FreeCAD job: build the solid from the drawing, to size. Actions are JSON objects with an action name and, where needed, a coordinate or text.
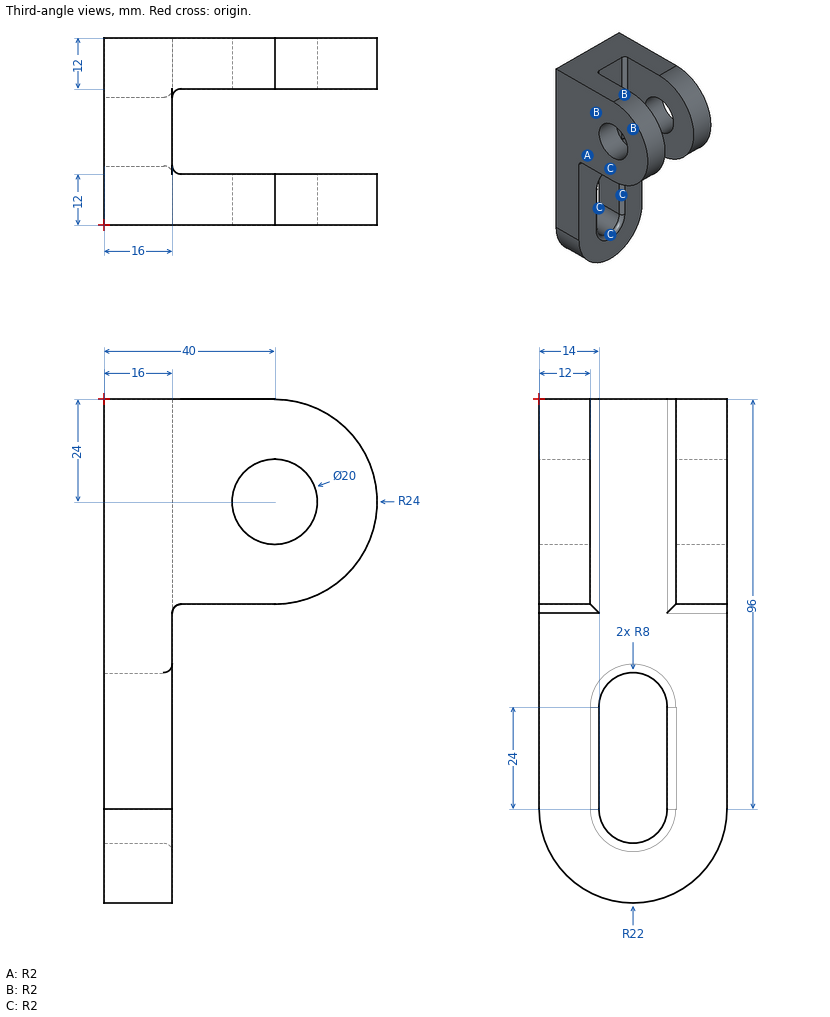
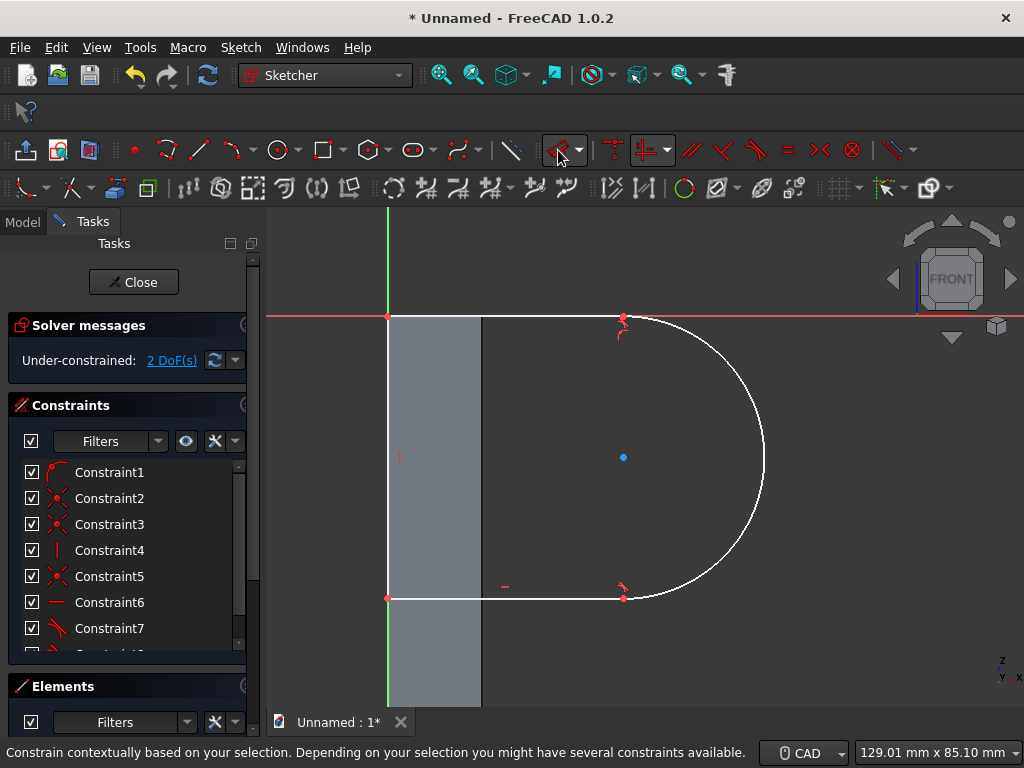
{"action": "left_click", "coordinate": [737, 541]}
{"action": "left_click", "coordinate": [763, 560]}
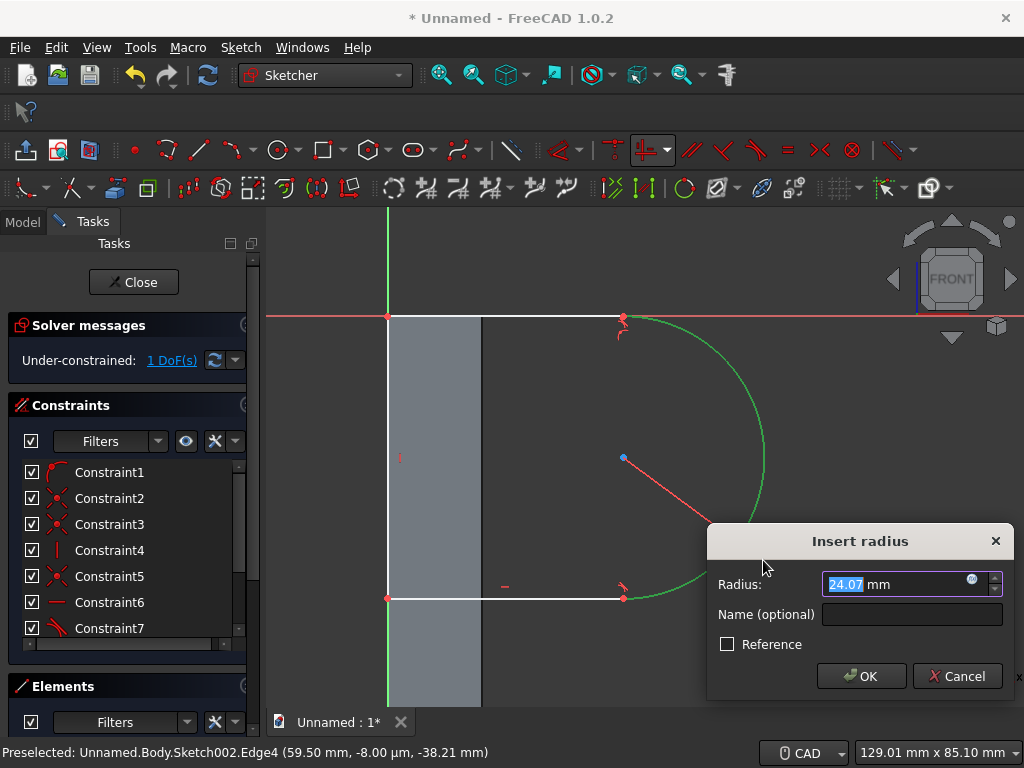
{"action": "type", "text": "24"}
{"action": "key", "text": "Return"}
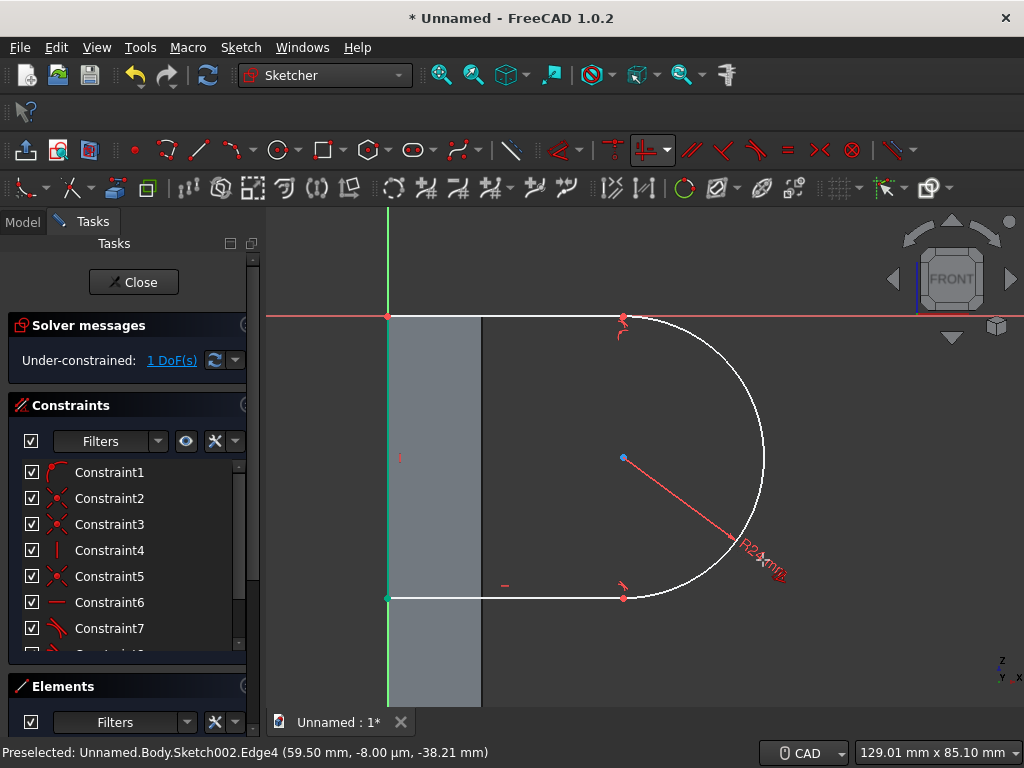
{"action": "left_click", "coordinate": [552, 316]}
{"action": "left_click", "coordinate": [505, 282]}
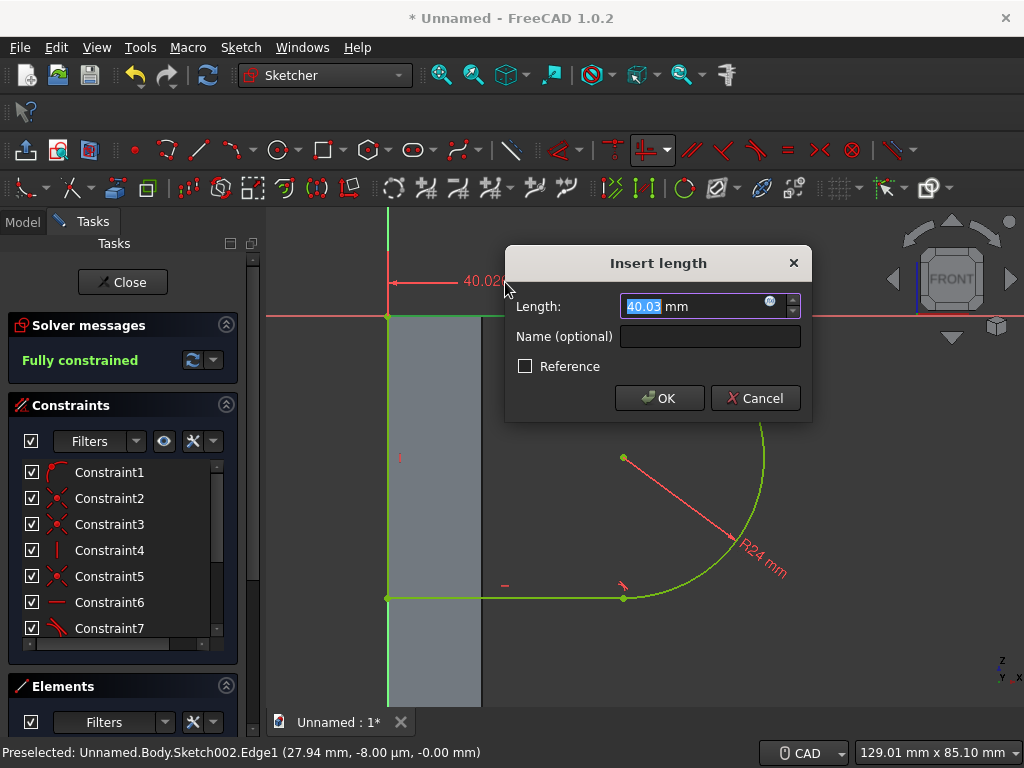
{"action": "type", "text": "40"}
{"action": "key", "text": "Return"}
{"action": "key", "text": "Escape"}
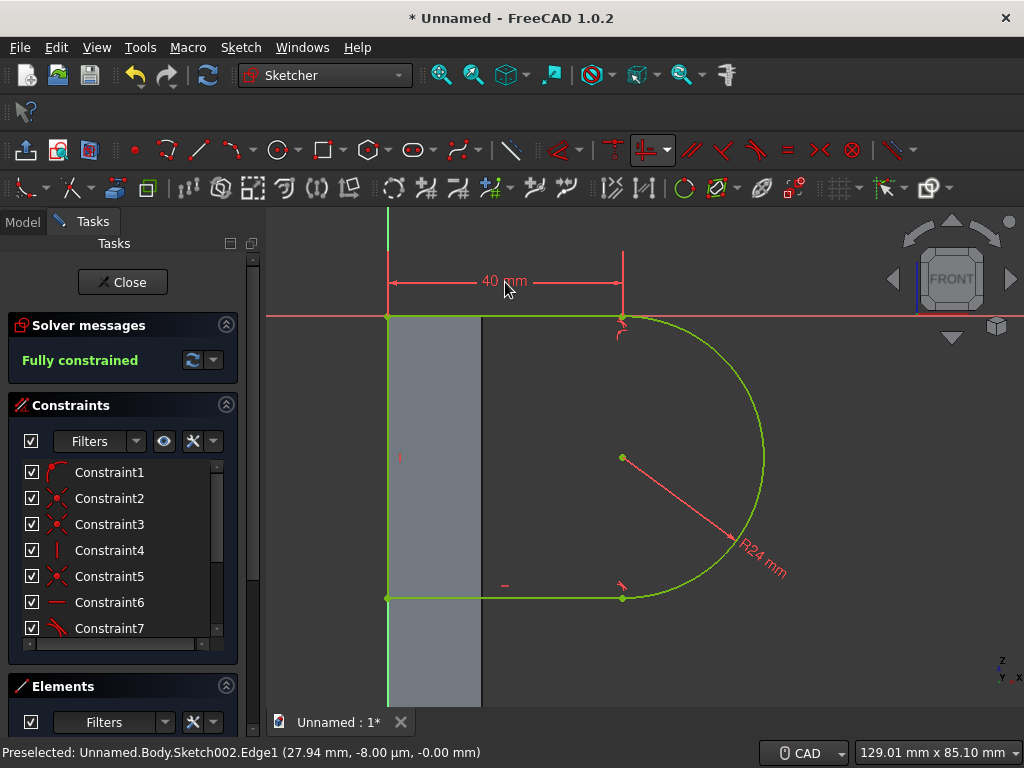
{"action": "left_click", "coordinate": [123, 282]}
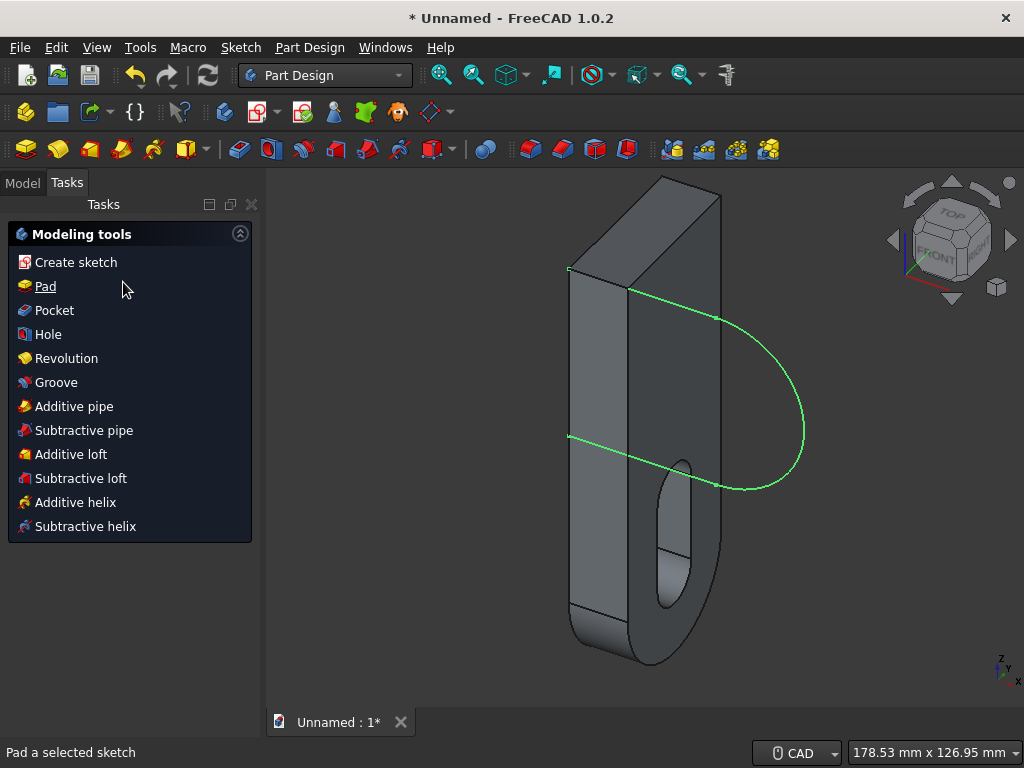
{"action": "left_click", "coordinate": [26, 150]}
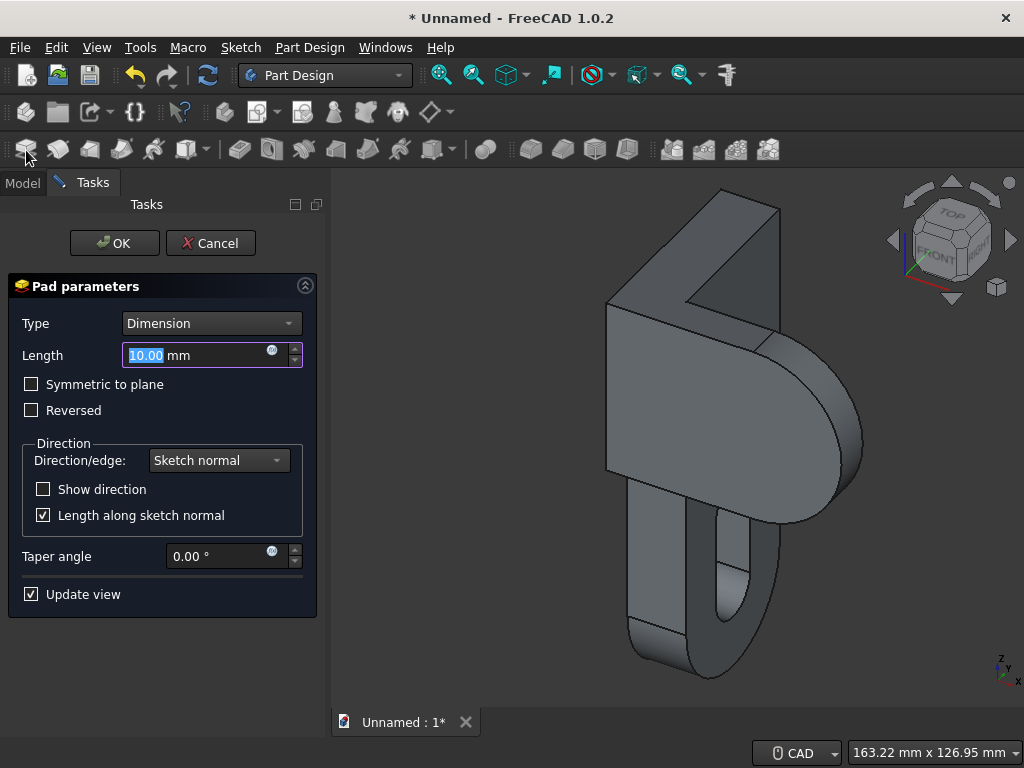
{"action": "type", "text": "12"}
{"action": "key", "text": "Tab"}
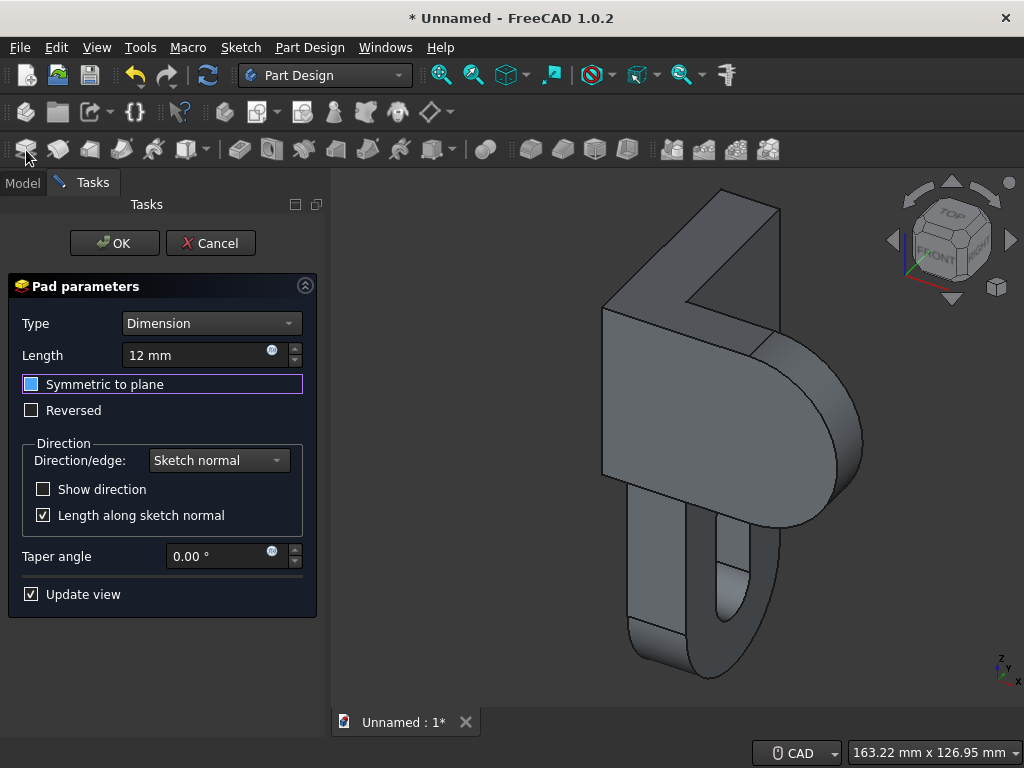
{"action": "left_click", "coordinate": [30, 410]}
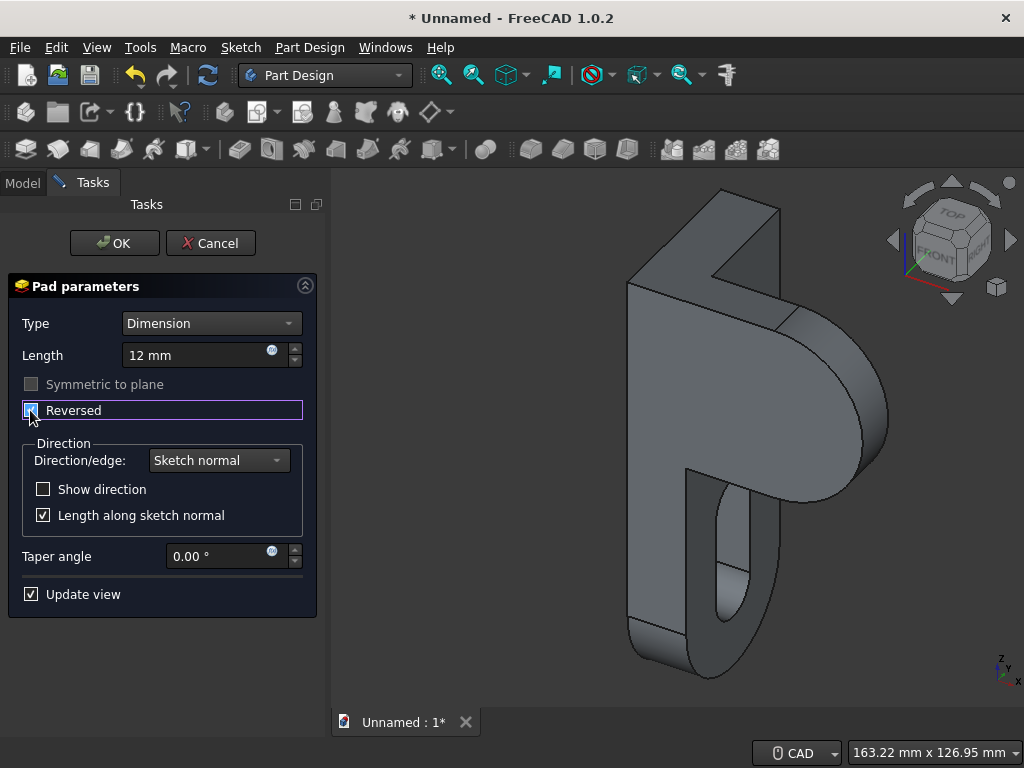
{"action": "left_click", "coordinate": [115, 243]}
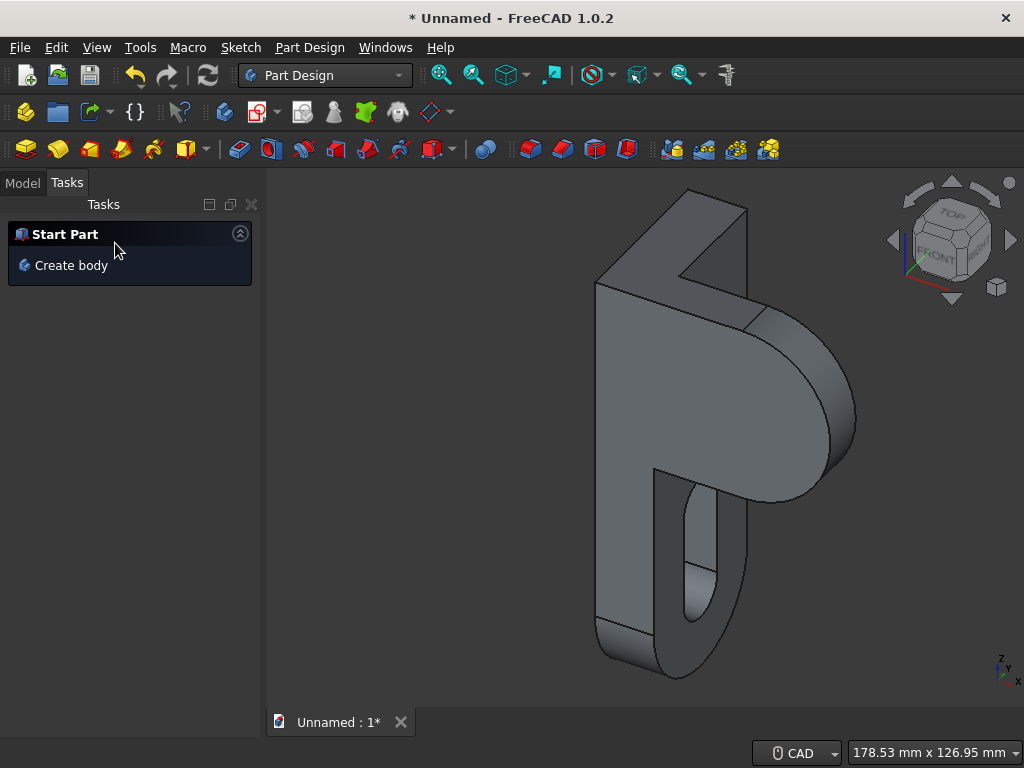
{"action": "left_click", "coordinate": [442, 76]}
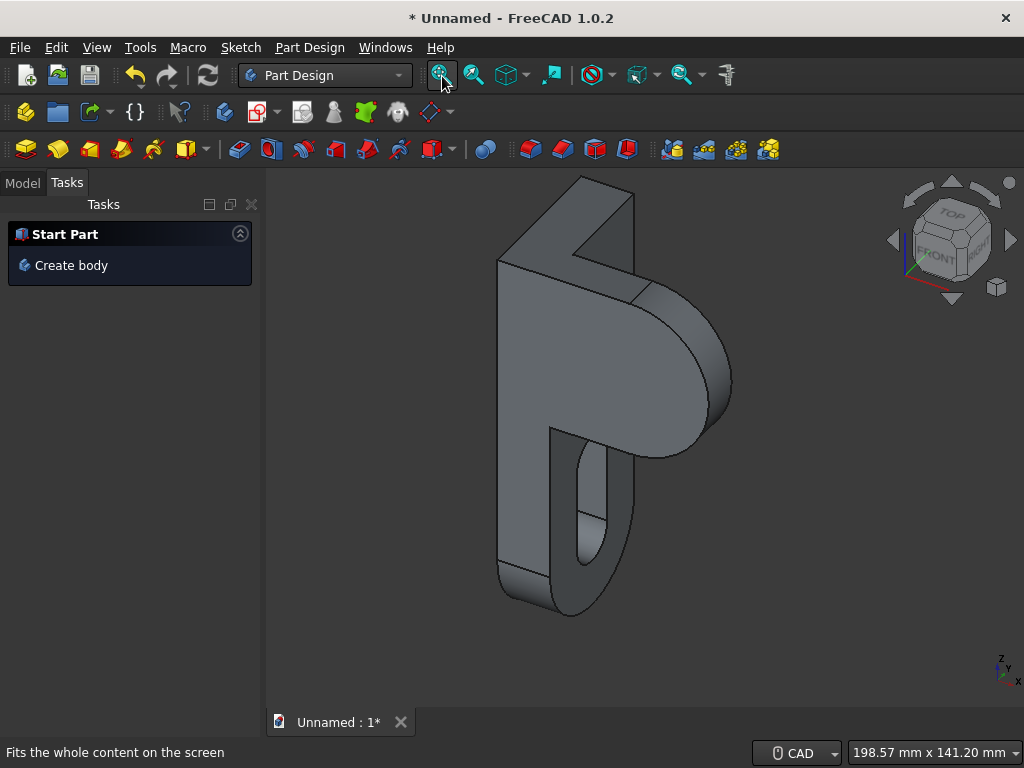
{"action": "left_click", "coordinate": [23, 182]}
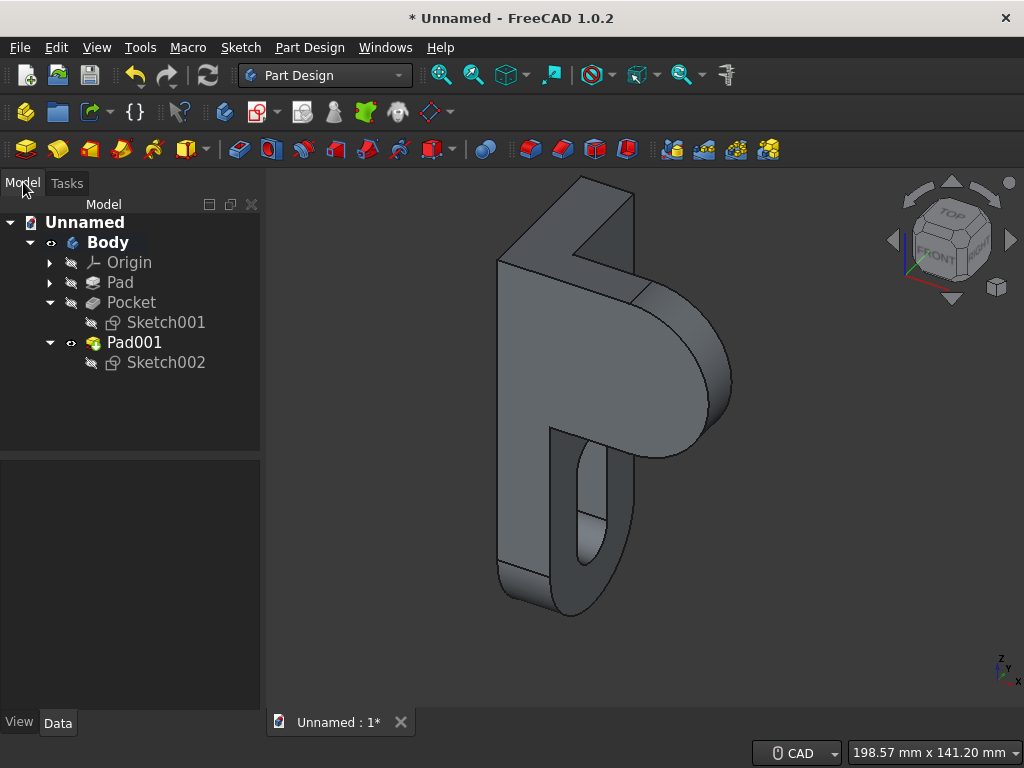
{"action": "left_click", "coordinate": [50, 263]}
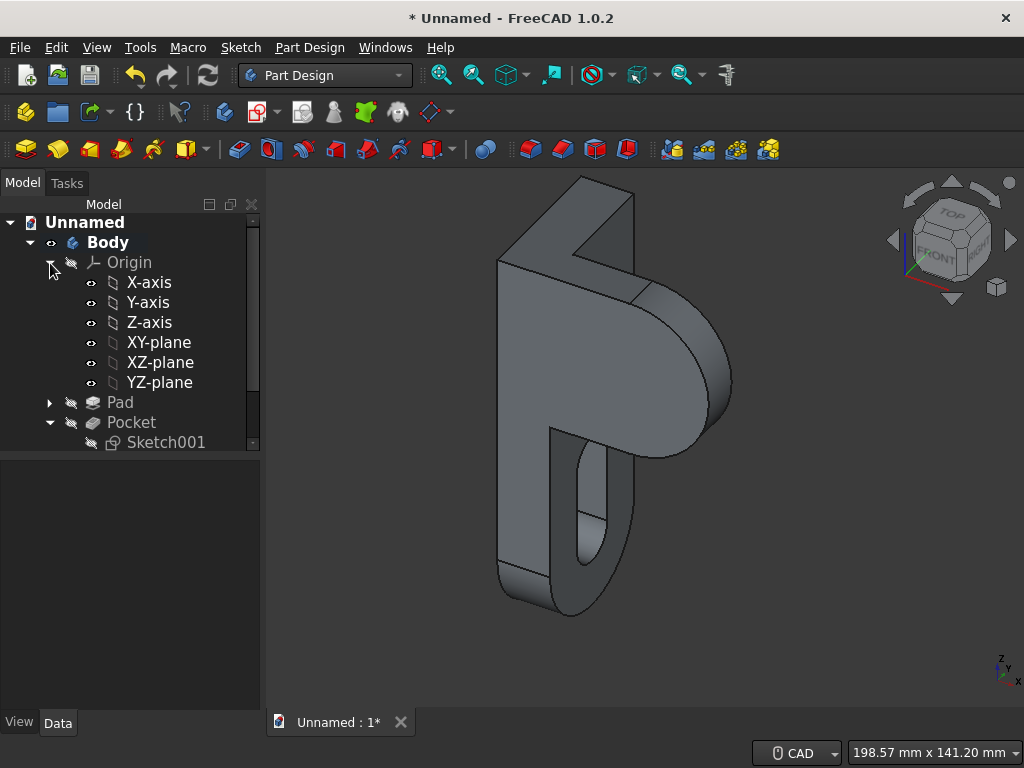
{"action": "left_click", "coordinate": [136, 363]}